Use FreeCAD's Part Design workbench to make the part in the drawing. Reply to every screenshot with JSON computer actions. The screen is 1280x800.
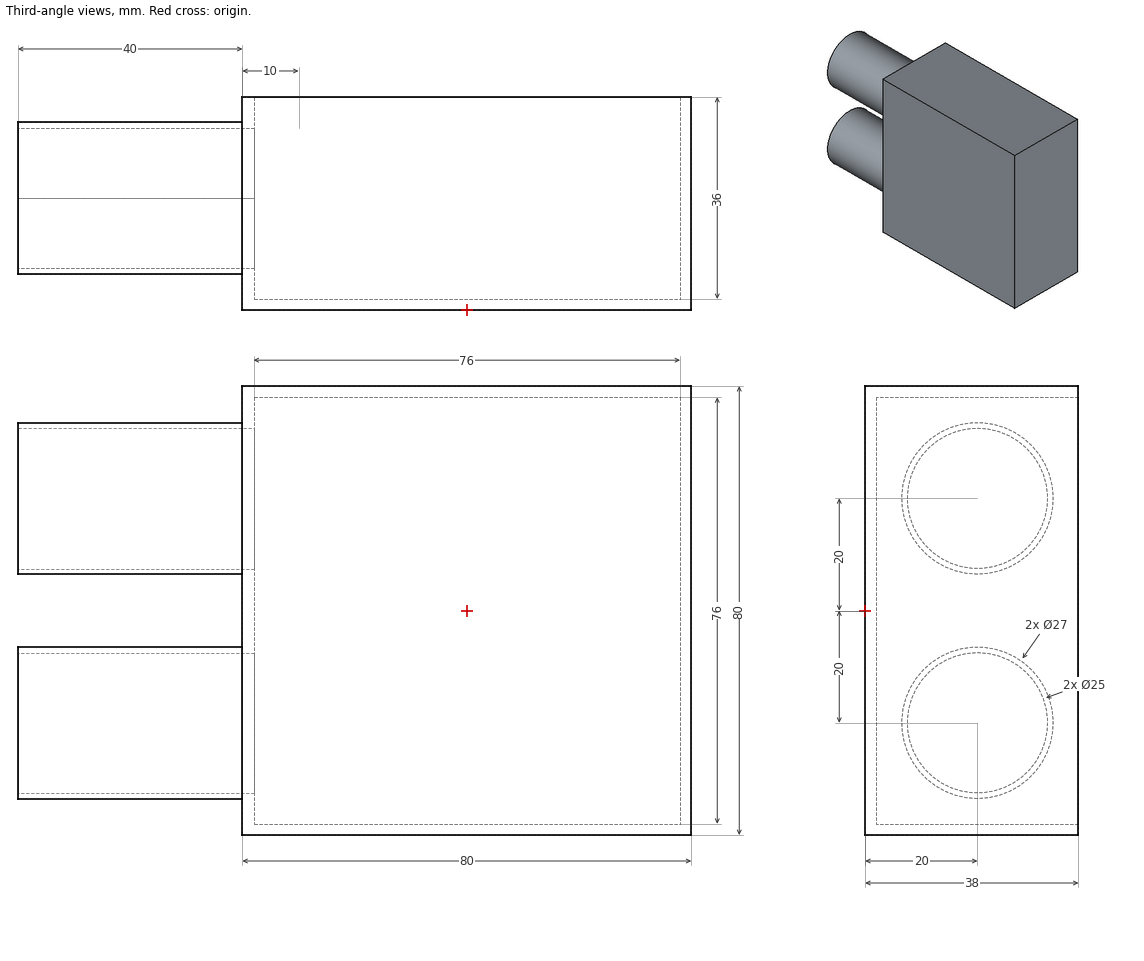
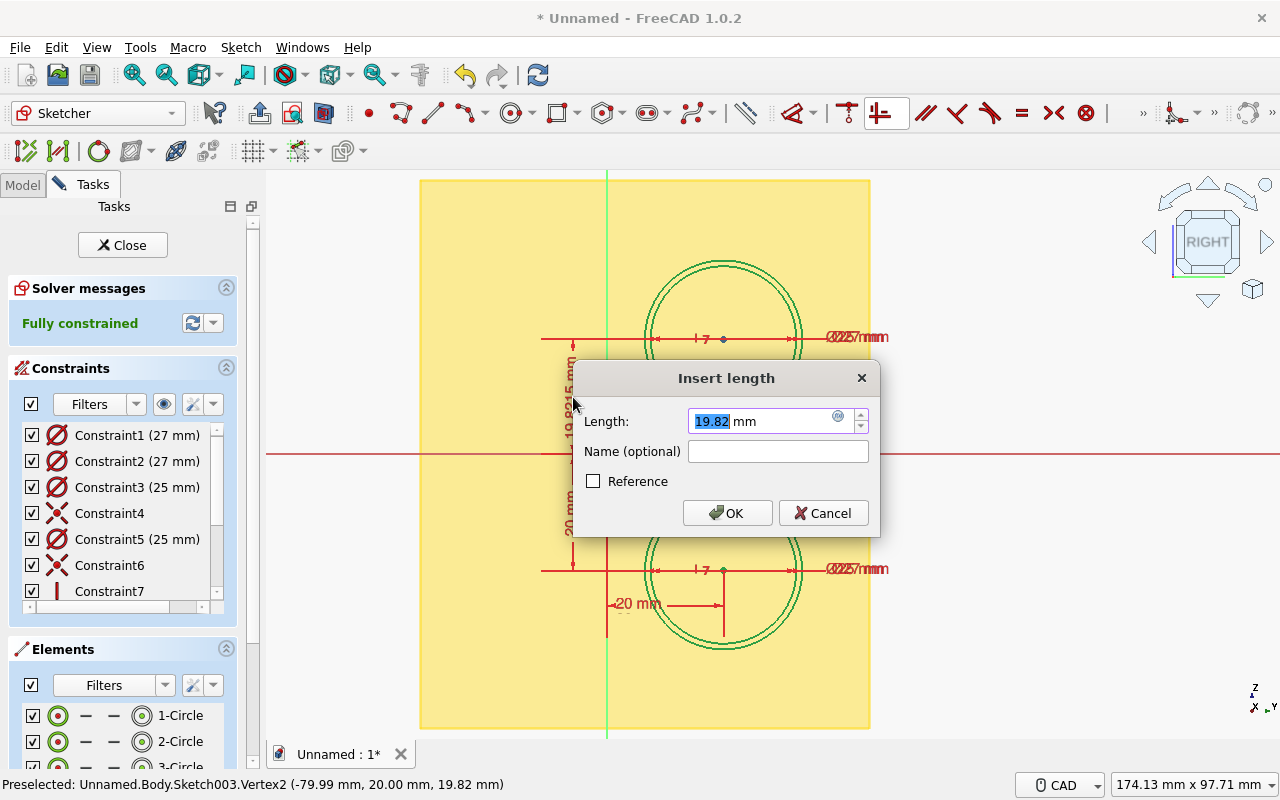
{"action": "type", "text": "20"}
{"action": "key", "text": "Return"}
{"action": "key", "text": "Escape"}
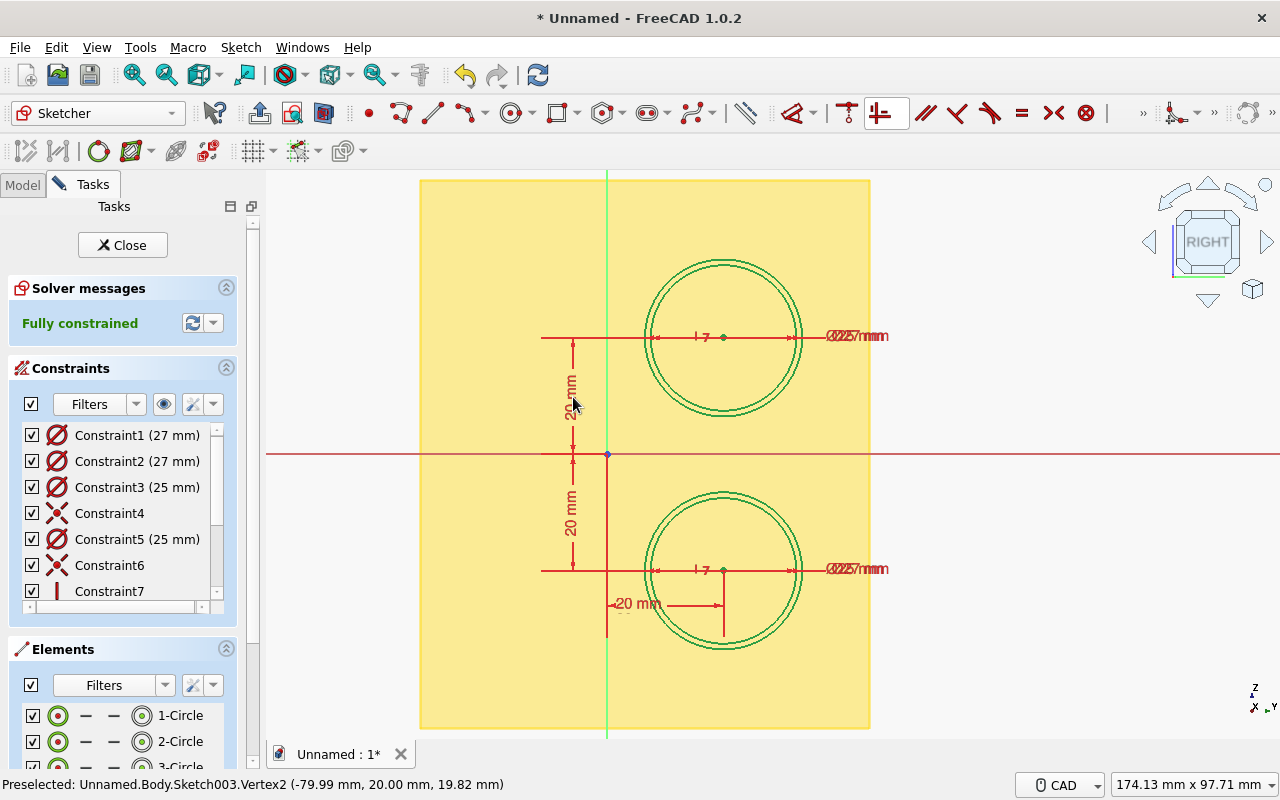
{"action": "left_click", "coordinate": [123, 245]}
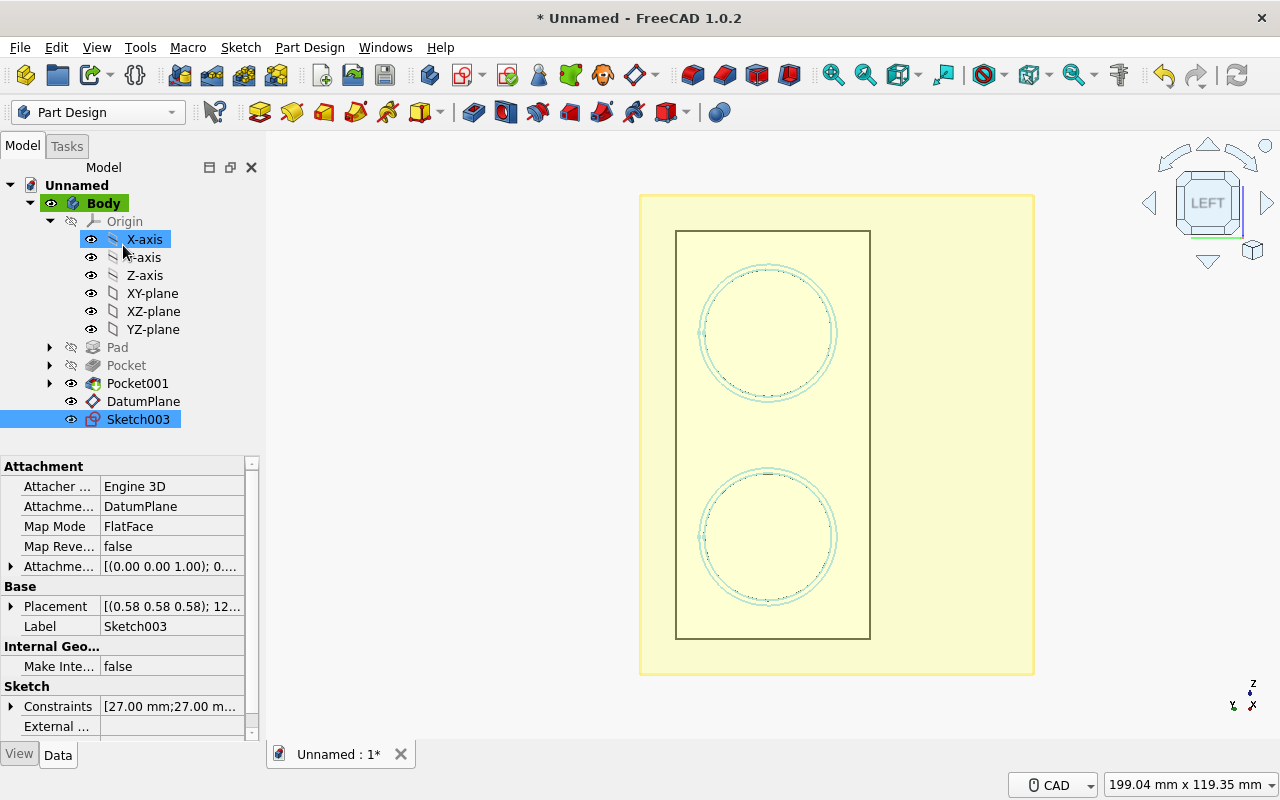
{"action": "left_click", "coordinate": [260, 112]}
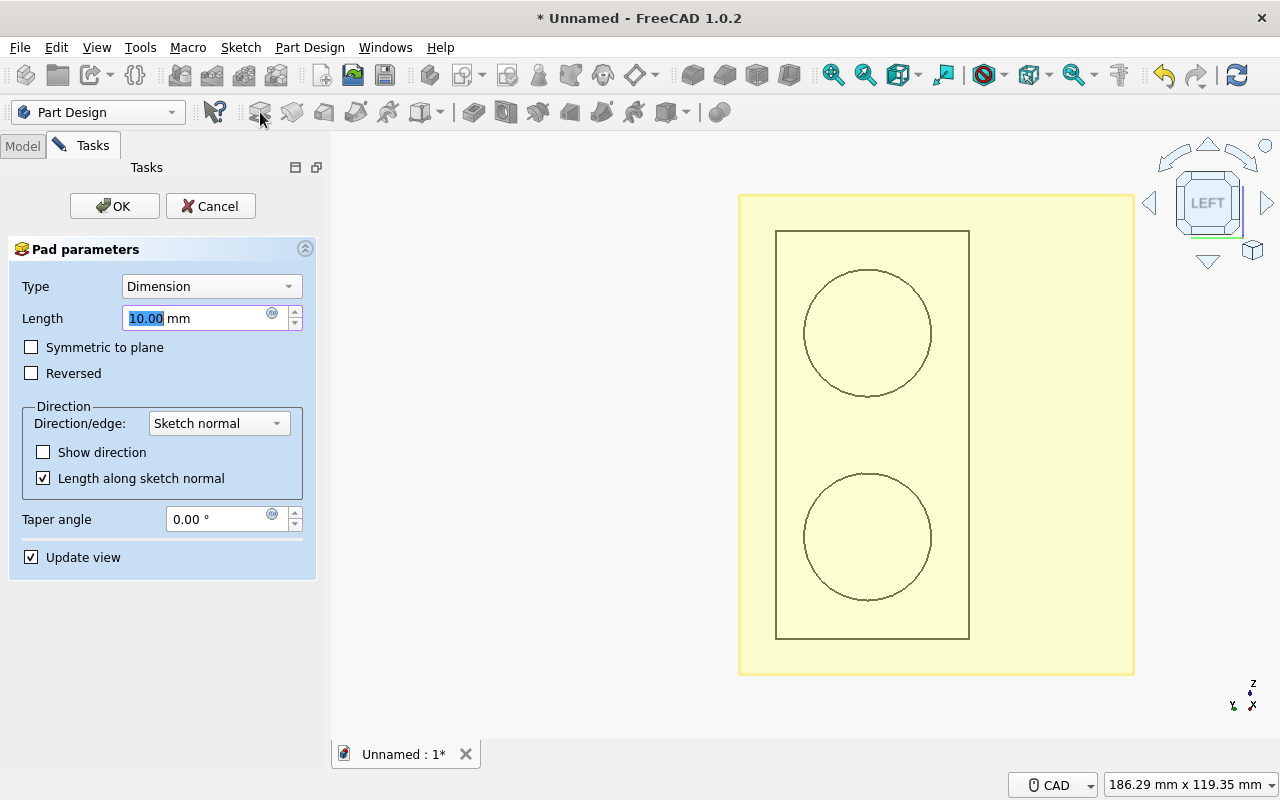
{"action": "type", "text": "40"}
{"action": "key", "text": "Tab"}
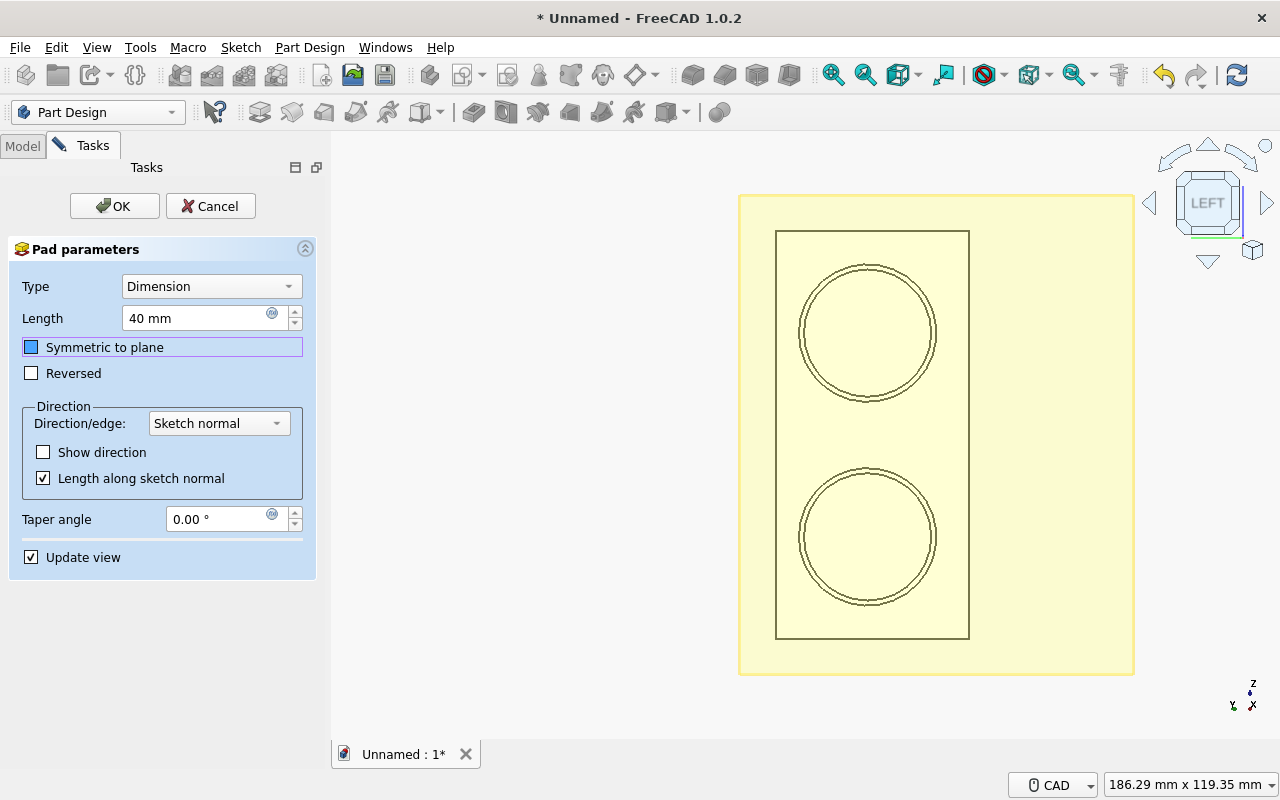
{"action": "left_click", "coordinate": [115, 206]}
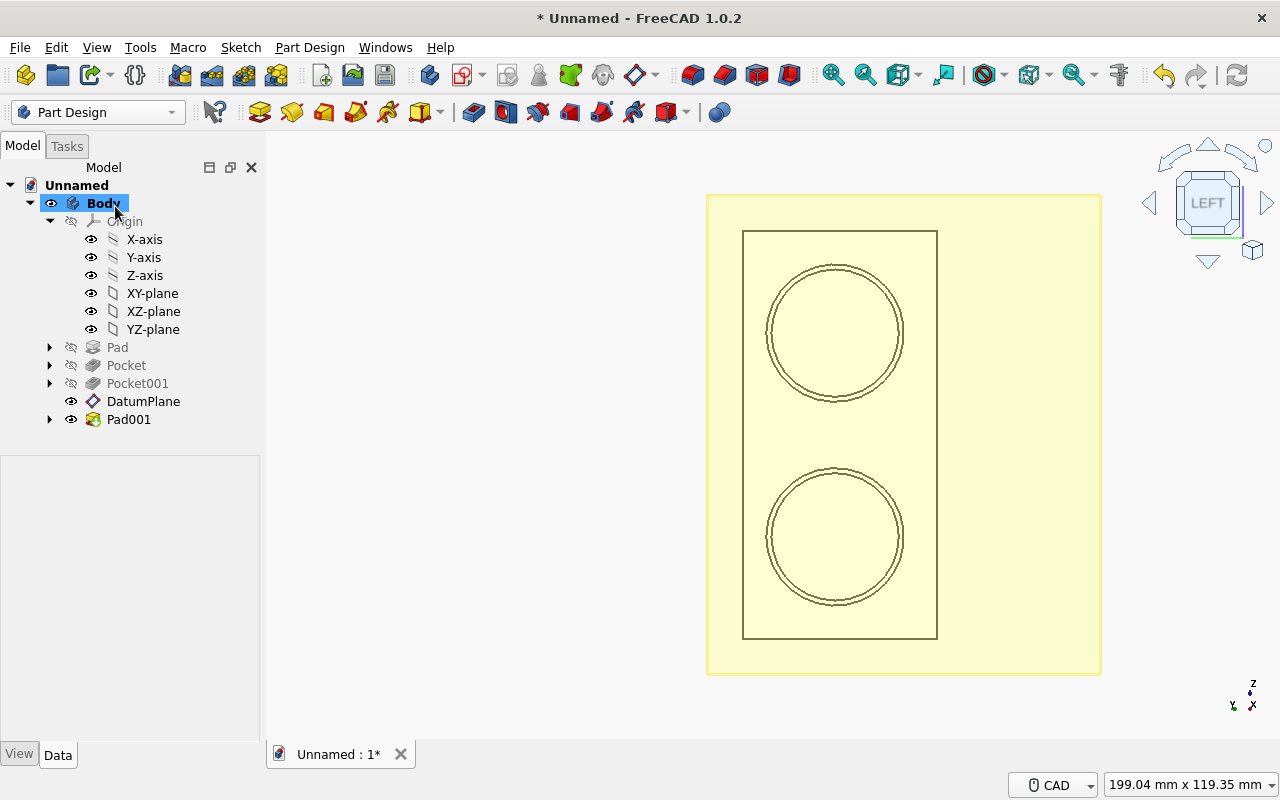
{"action": "left_click", "coordinate": [116, 401]}
{"action": "key", "text": "space"}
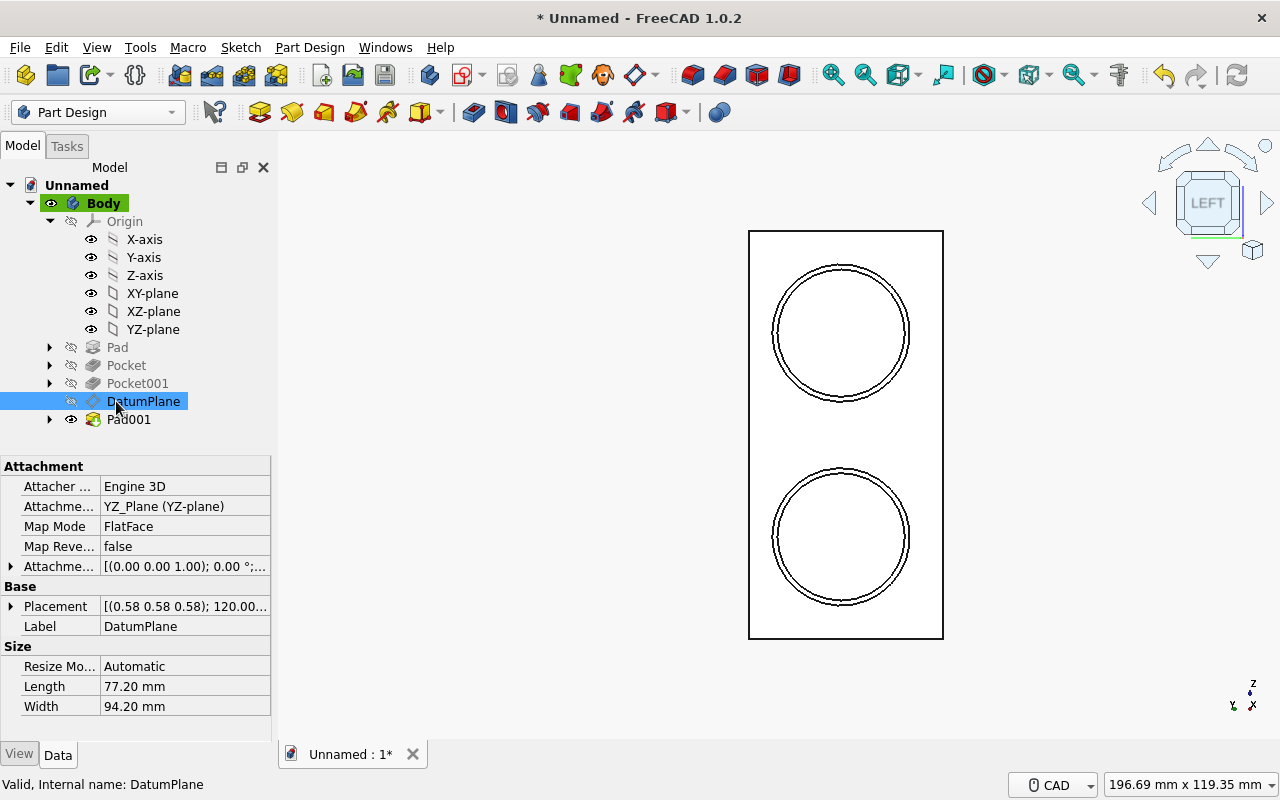
{"action": "key", "text": "0"}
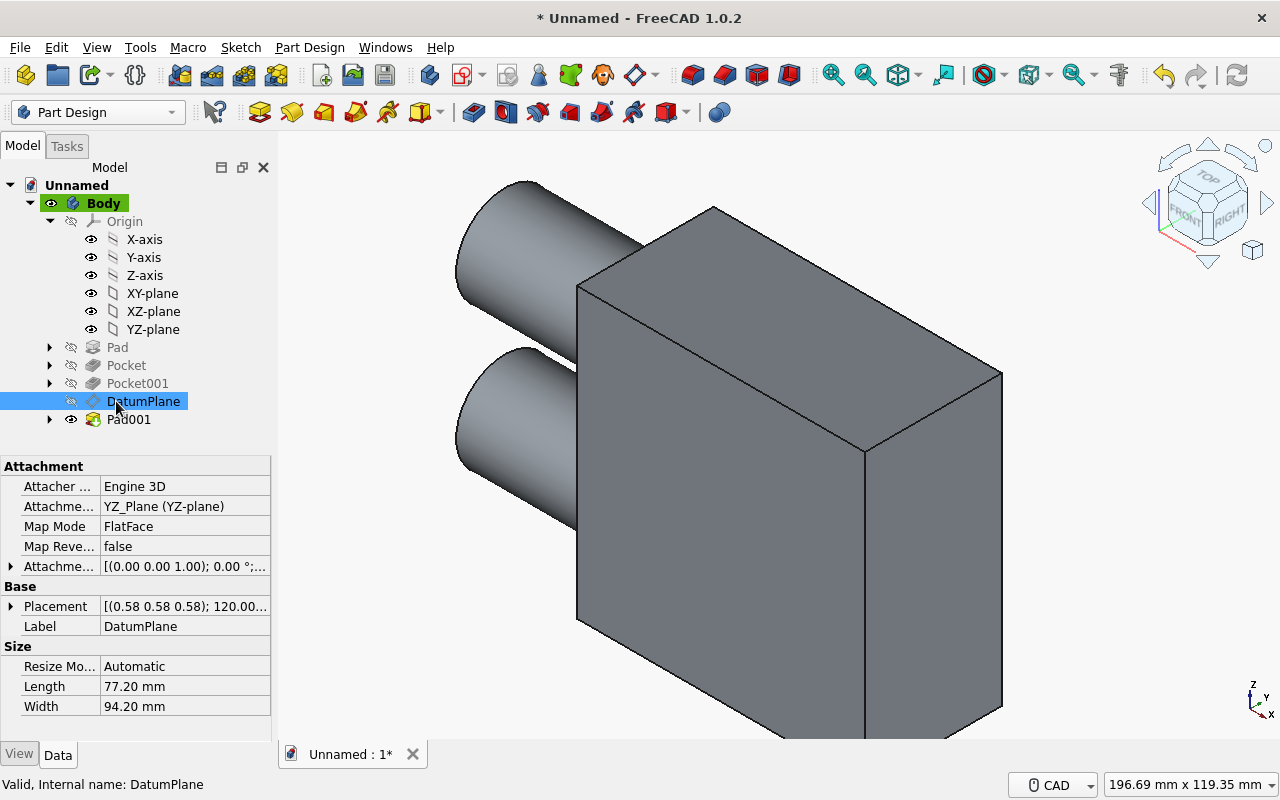
{"action": "left_click", "coordinate": [834, 76]}